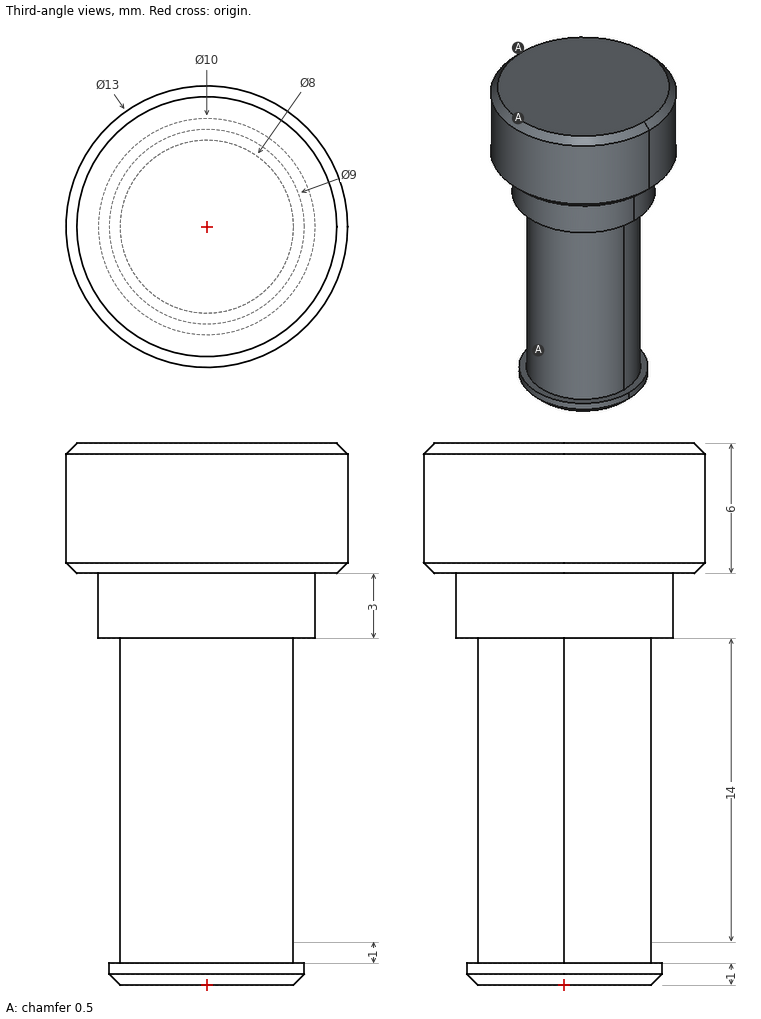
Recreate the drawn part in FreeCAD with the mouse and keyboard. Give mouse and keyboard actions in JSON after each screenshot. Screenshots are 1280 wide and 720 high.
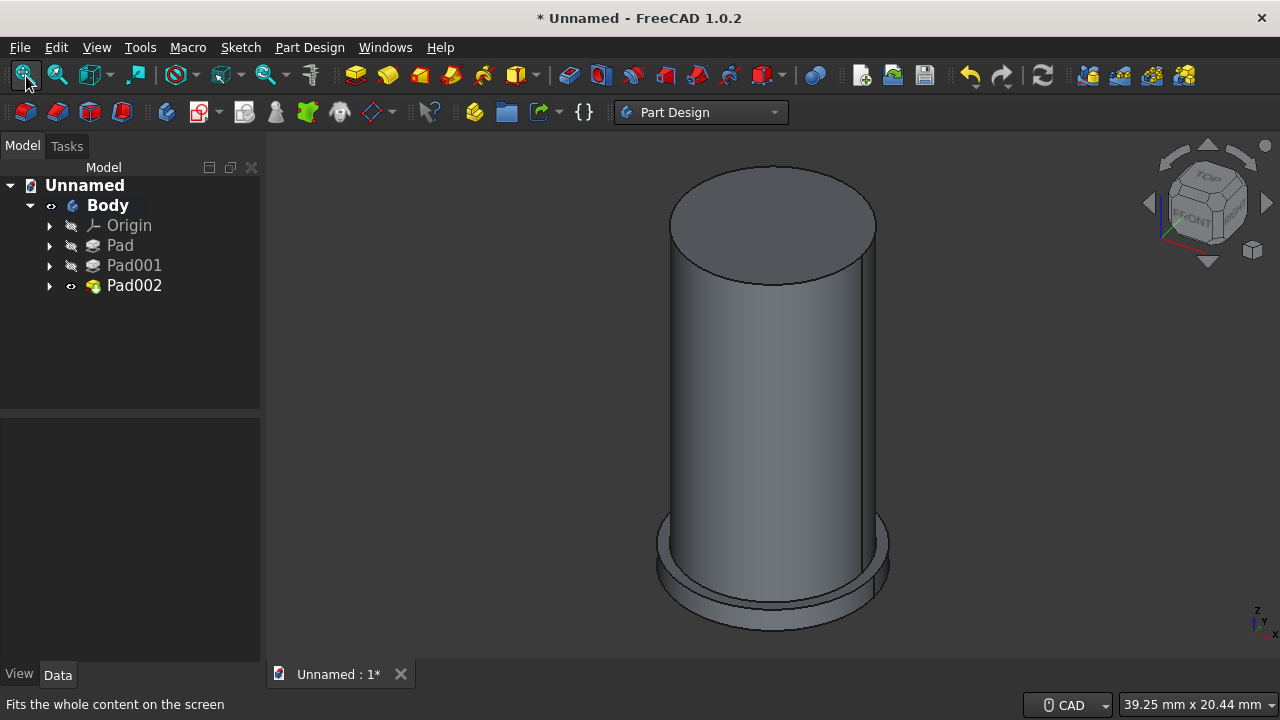
{"action": "left_click", "coordinate": [773, 225]}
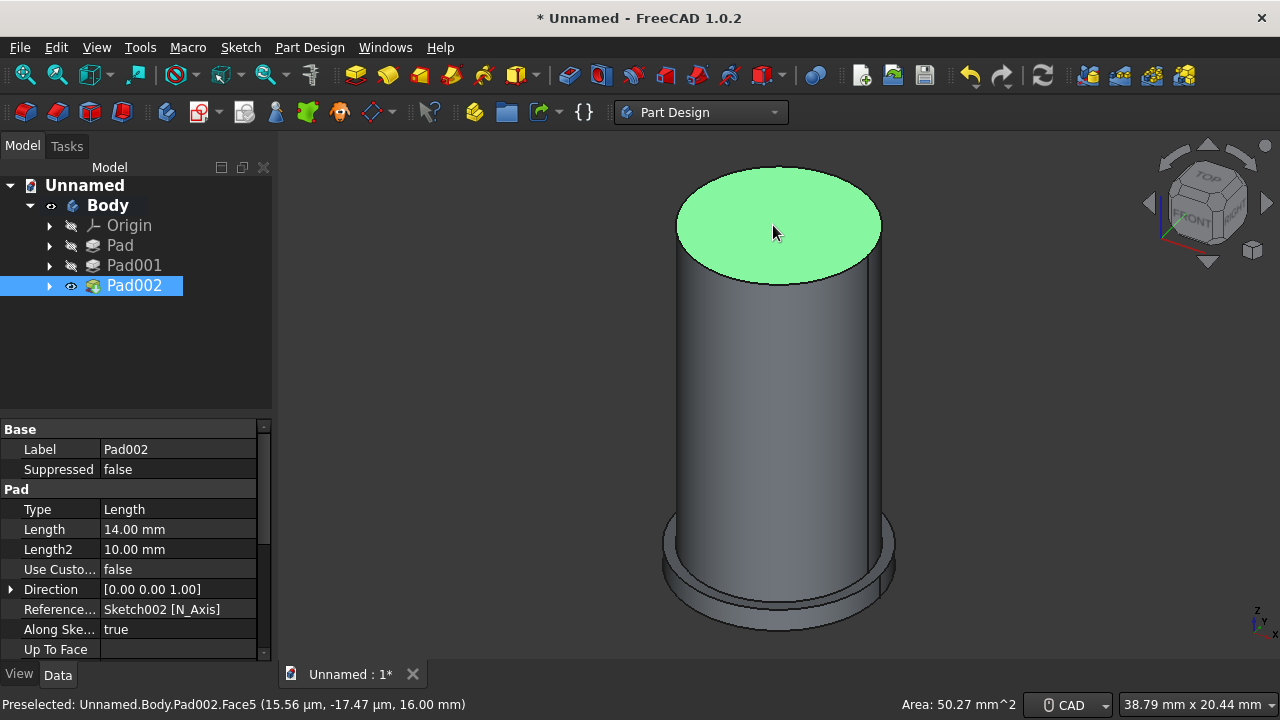
{"action": "left_click", "coordinate": [200, 112]}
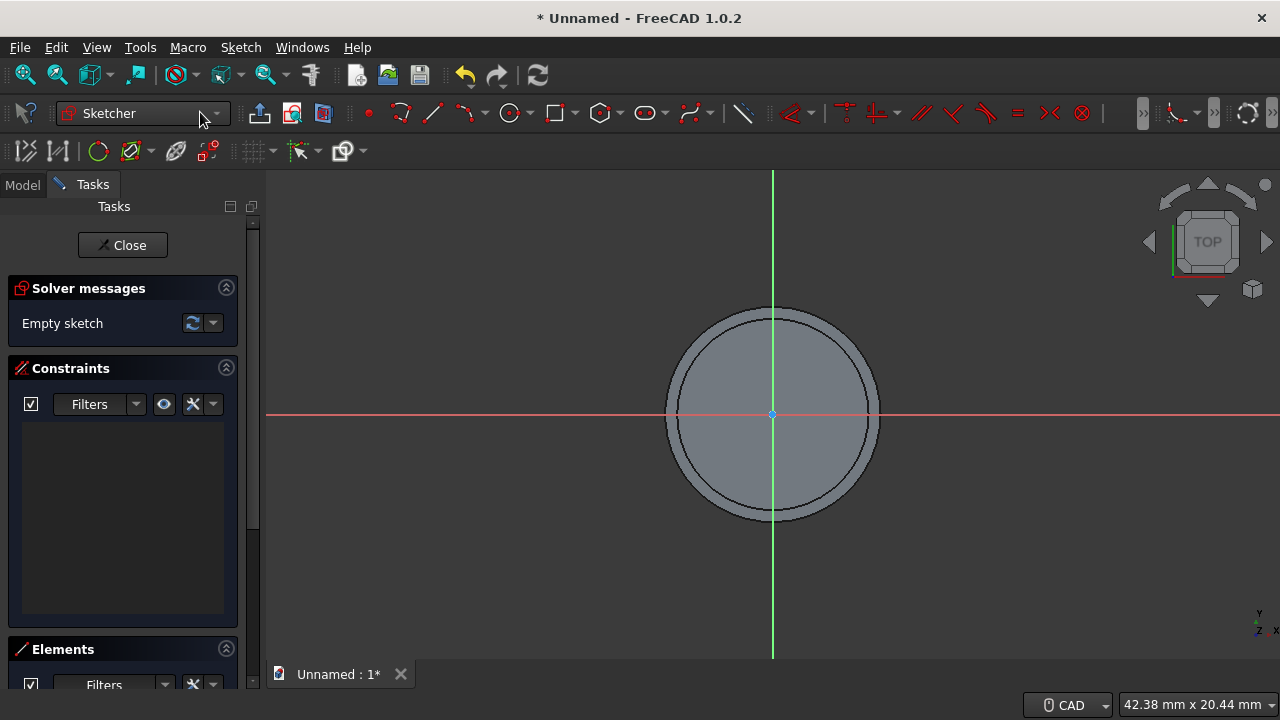
{"action": "left_click", "coordinate": [510, 114]}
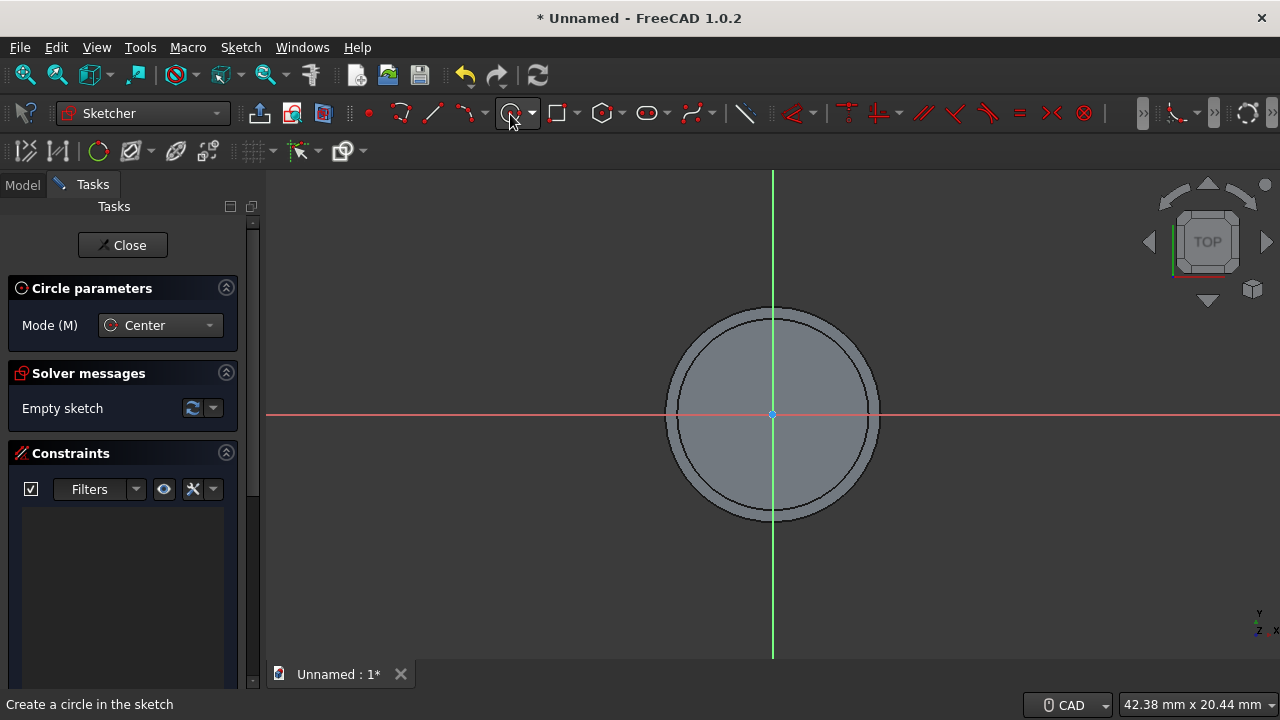
{"action": "left_click", "coordinate": [773, 414]}
{"action": "mouse_move", "coordinate": [857, 330]}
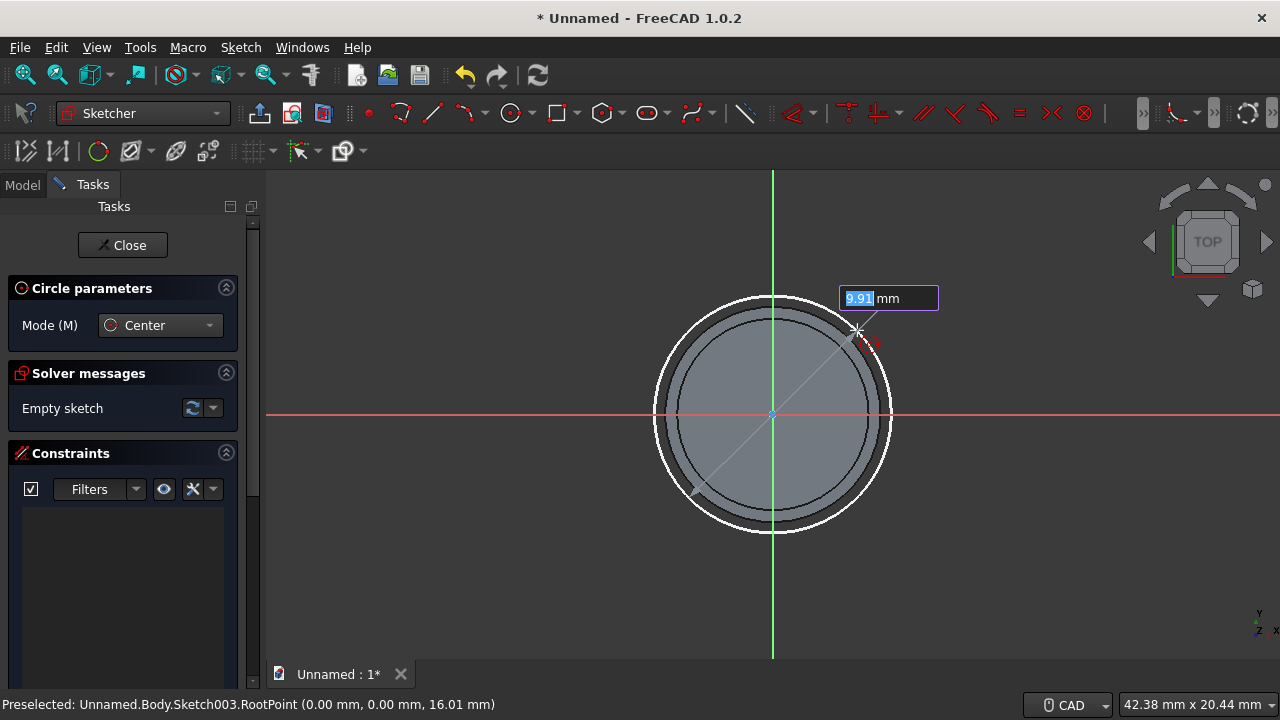
{"action": "type", "text": "10"}
{"action": "key", "text": "Return"}
{"action": "key", "text": "Escape"}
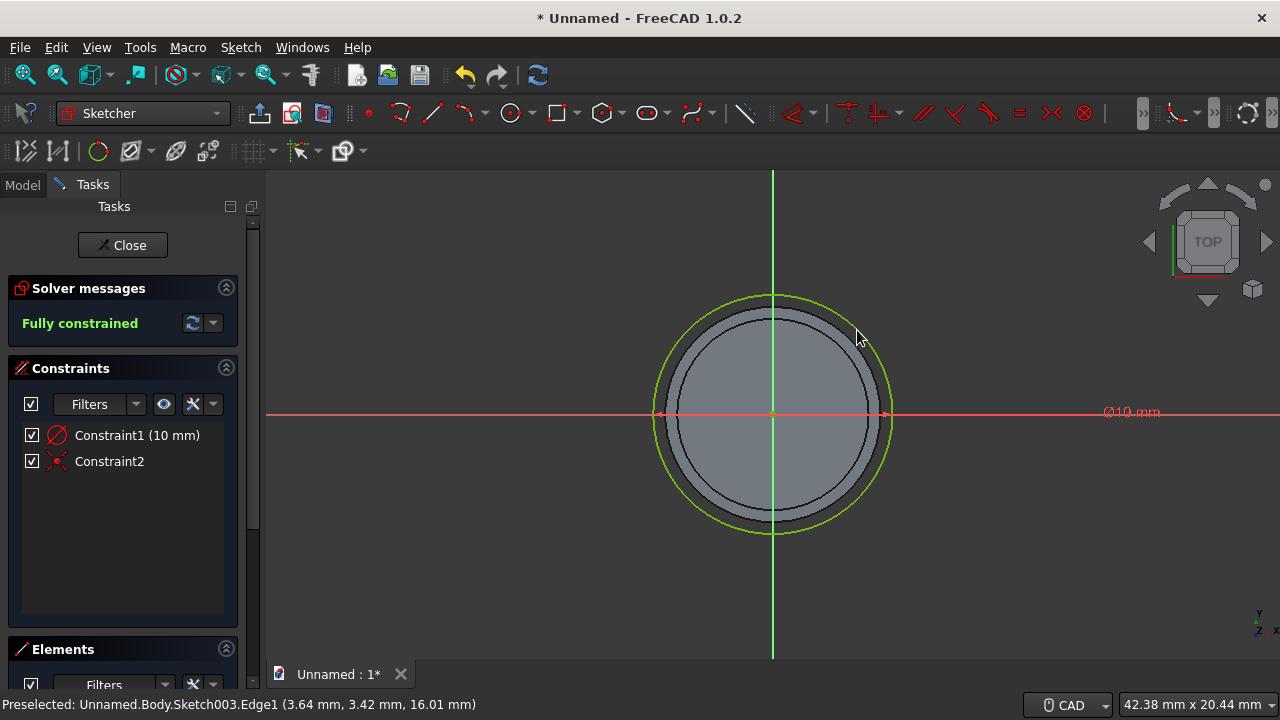
{"action": "left_click", "coordinate": [123, 245]}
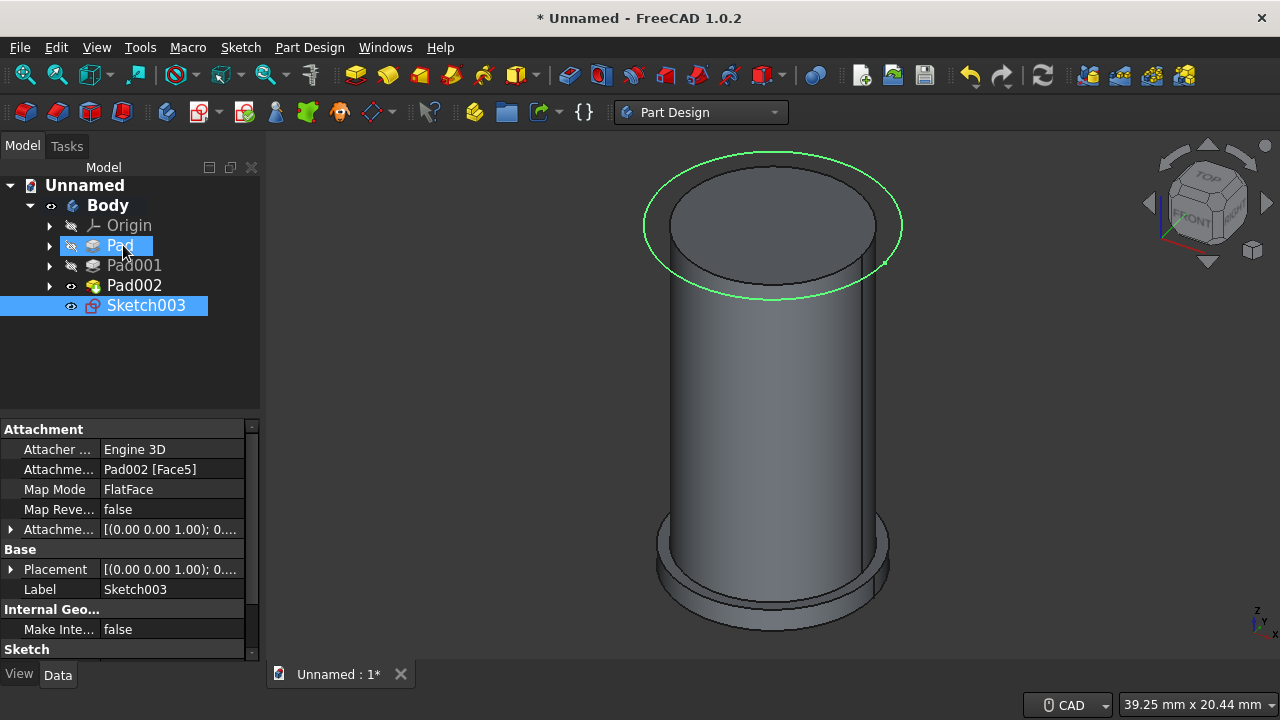
{"action": "left_click", "coordinate": [356, 76]}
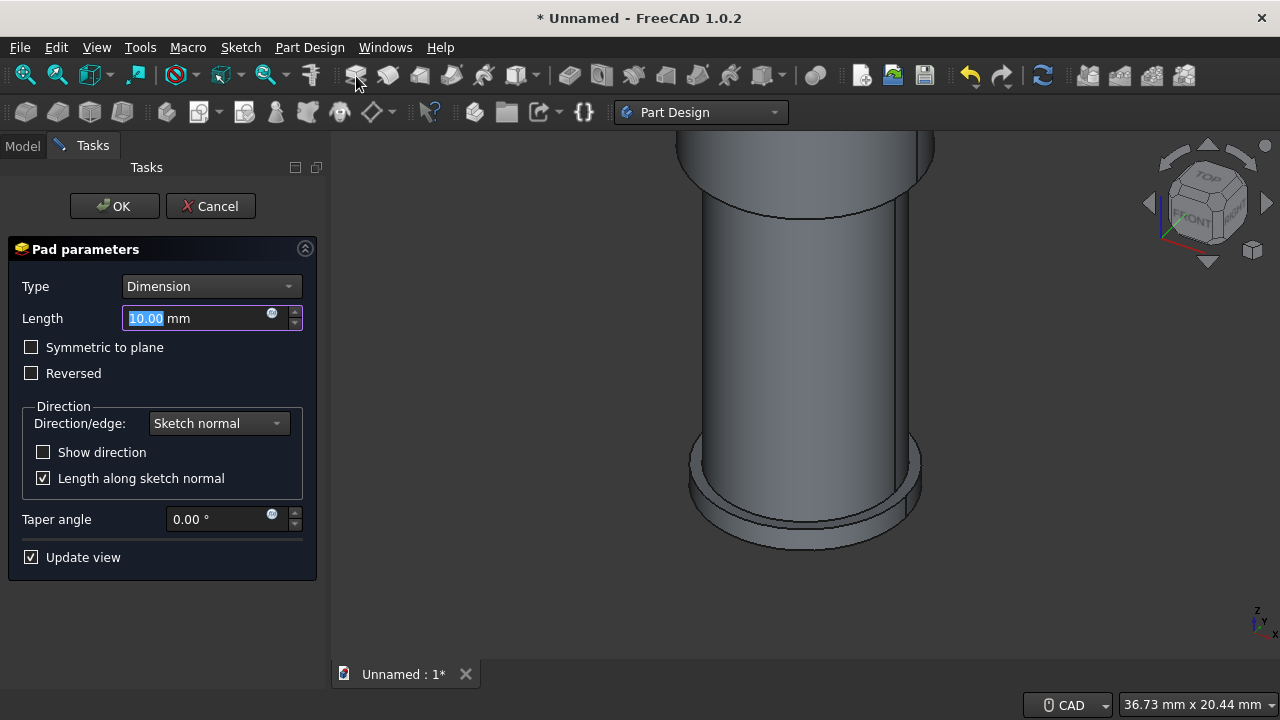
{"action": "type", "text": "3"}
{"action": "key", "text": "Tab"}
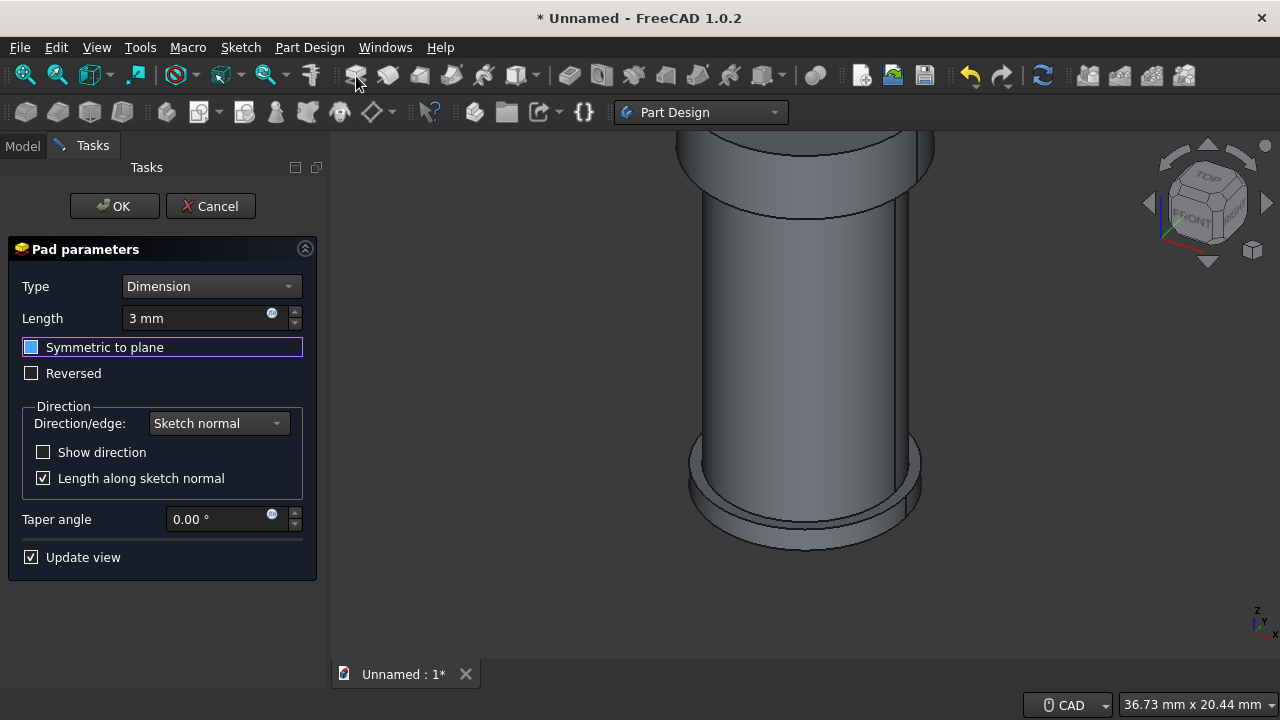
{"action": "left_click", "coordinate": [115, 206]}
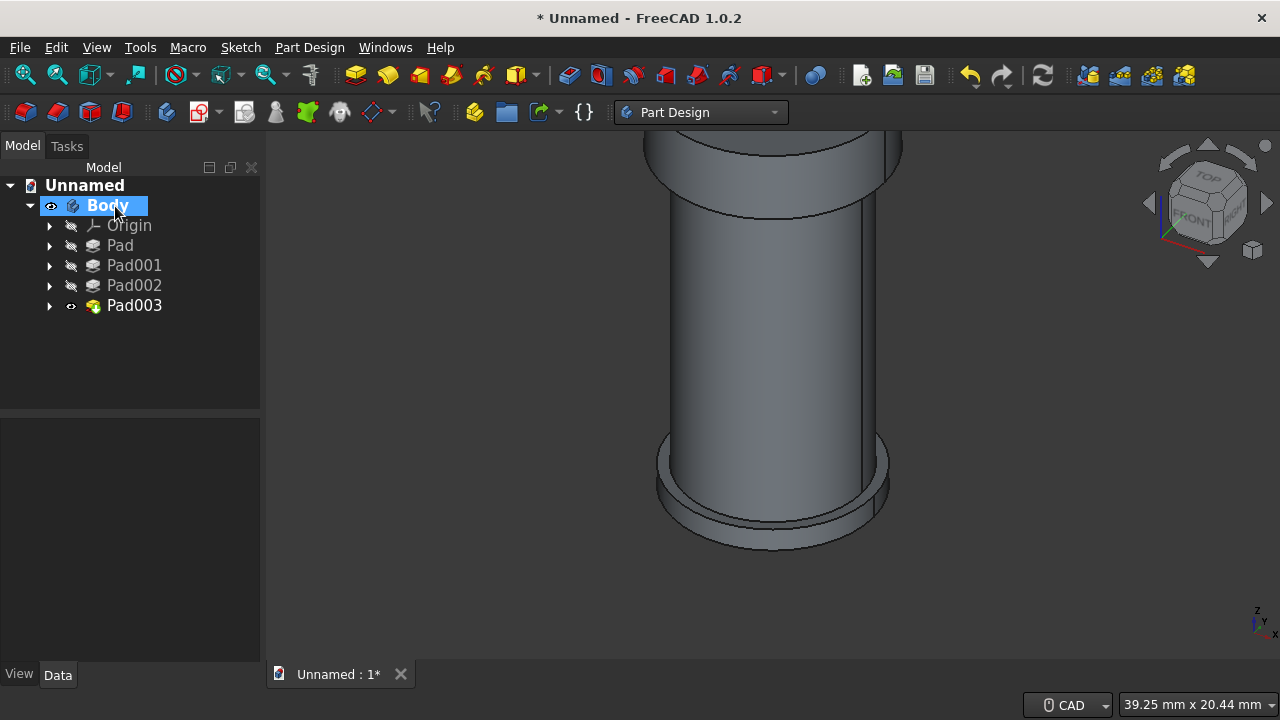
{"action": "left_click", "coordinate": [26, 76]}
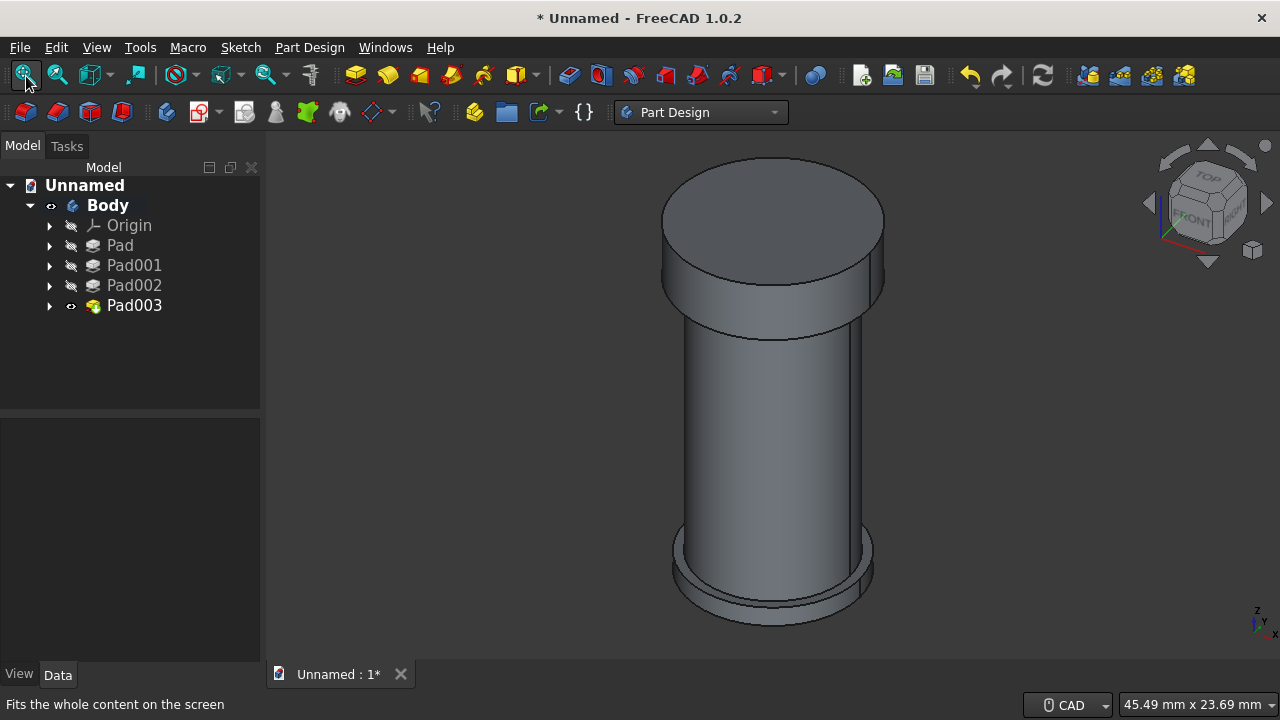
{"action": "left_click", "coordinate": [773, 221]}